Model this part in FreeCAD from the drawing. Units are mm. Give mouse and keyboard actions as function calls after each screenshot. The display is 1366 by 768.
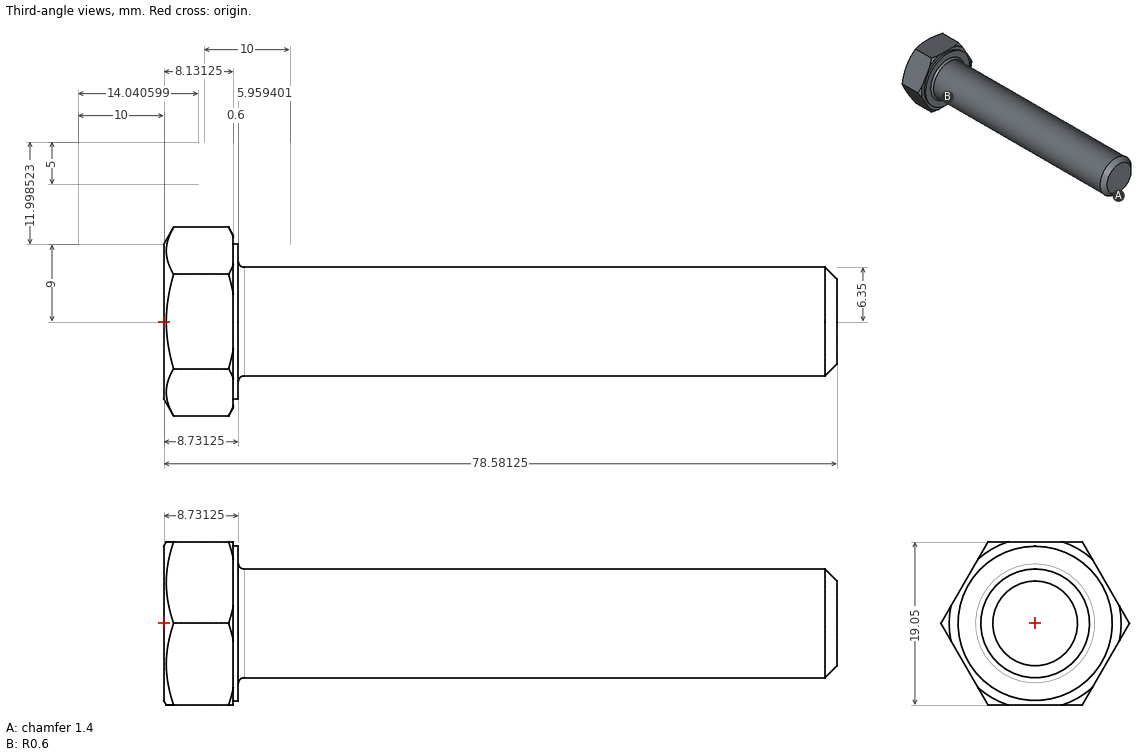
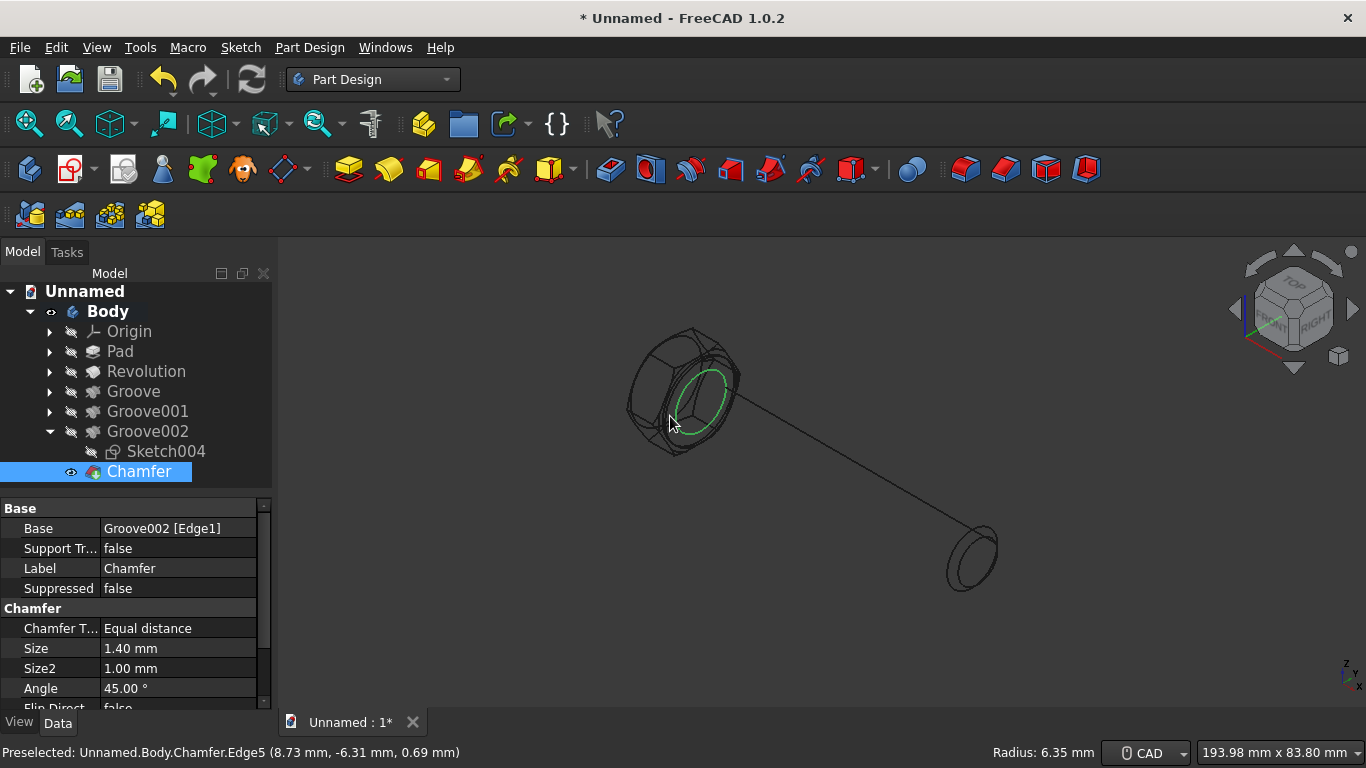
key(v)
key(1)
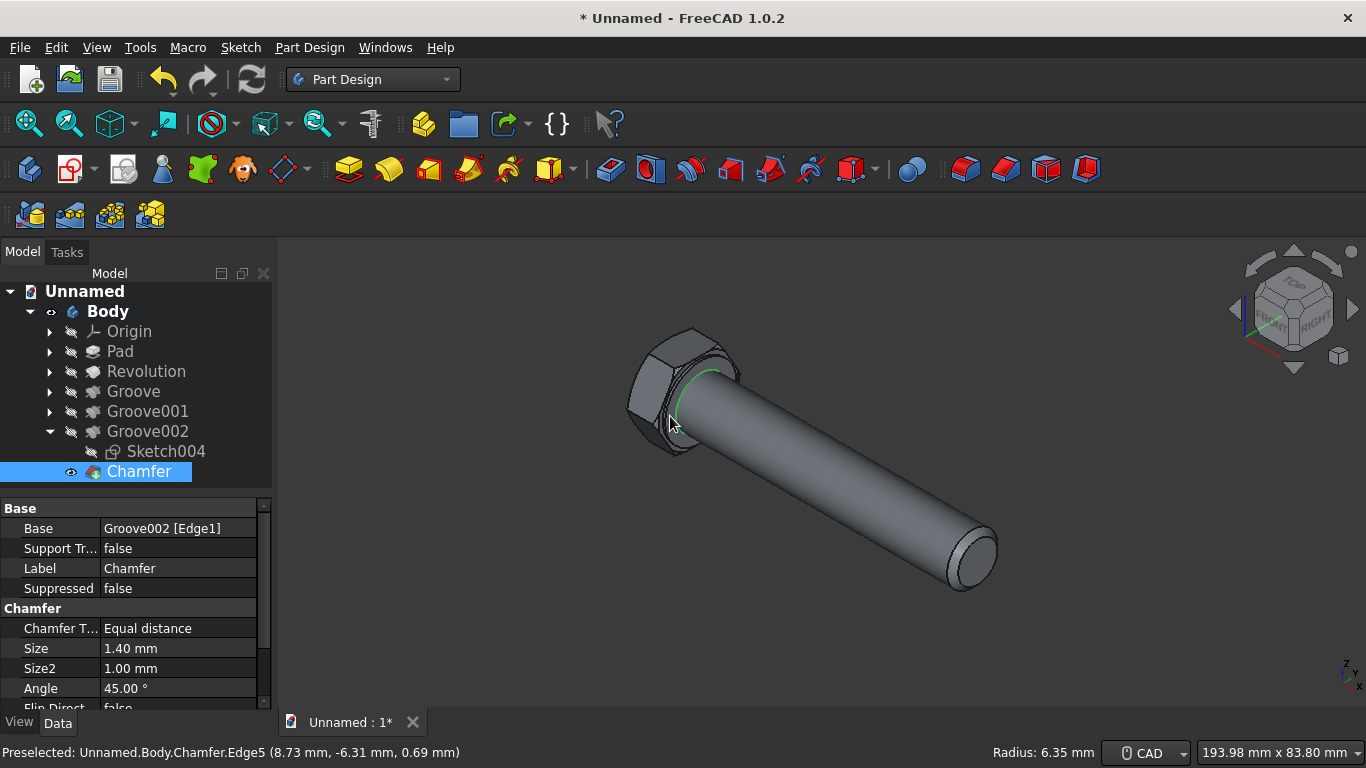
click(966, 170)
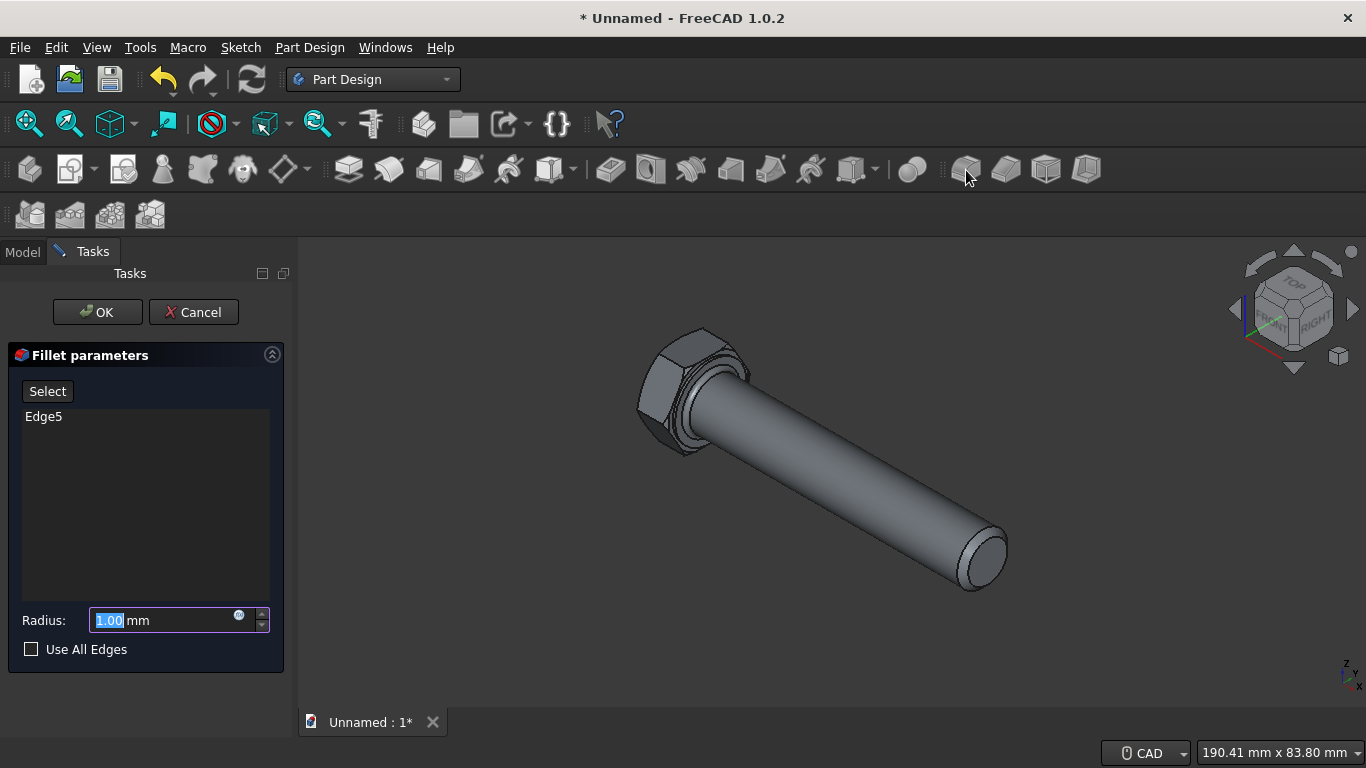
text(0.6)
key(Tab)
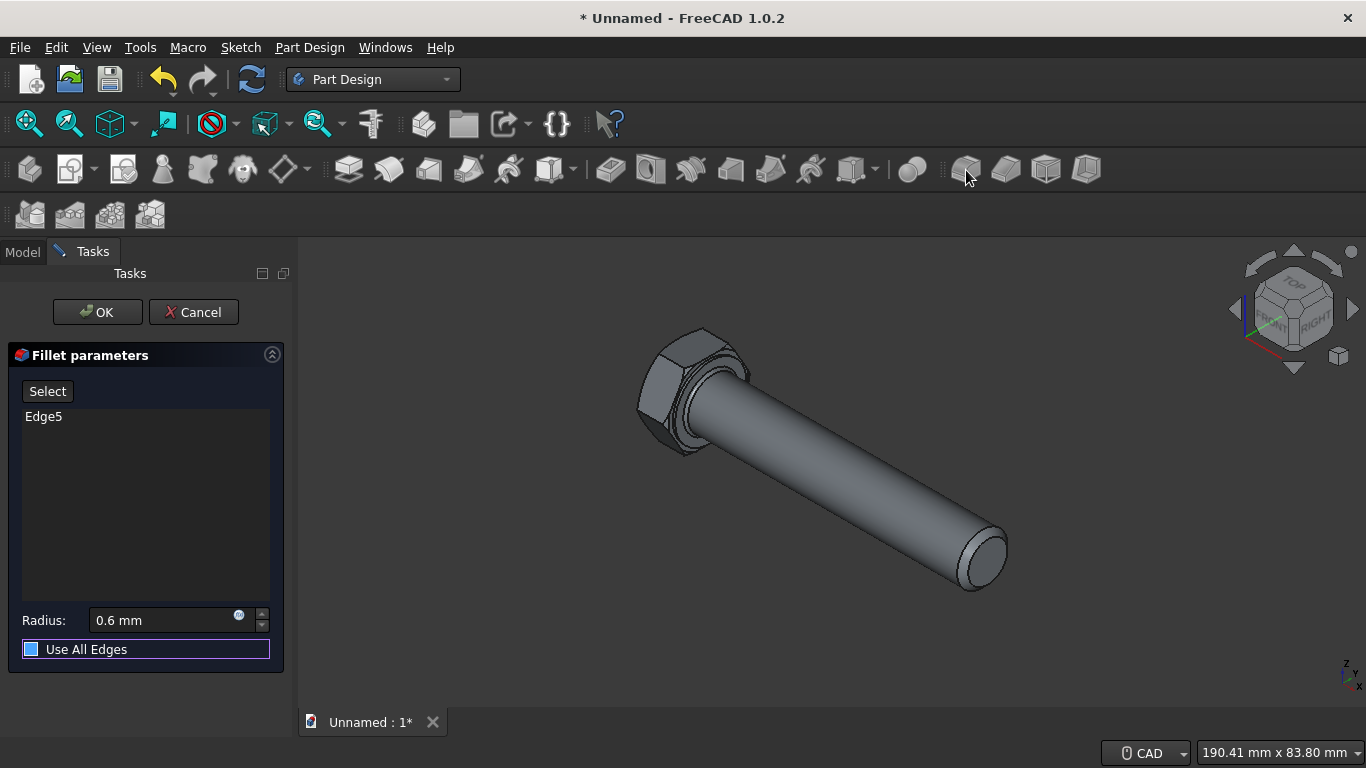
click(98, 312)